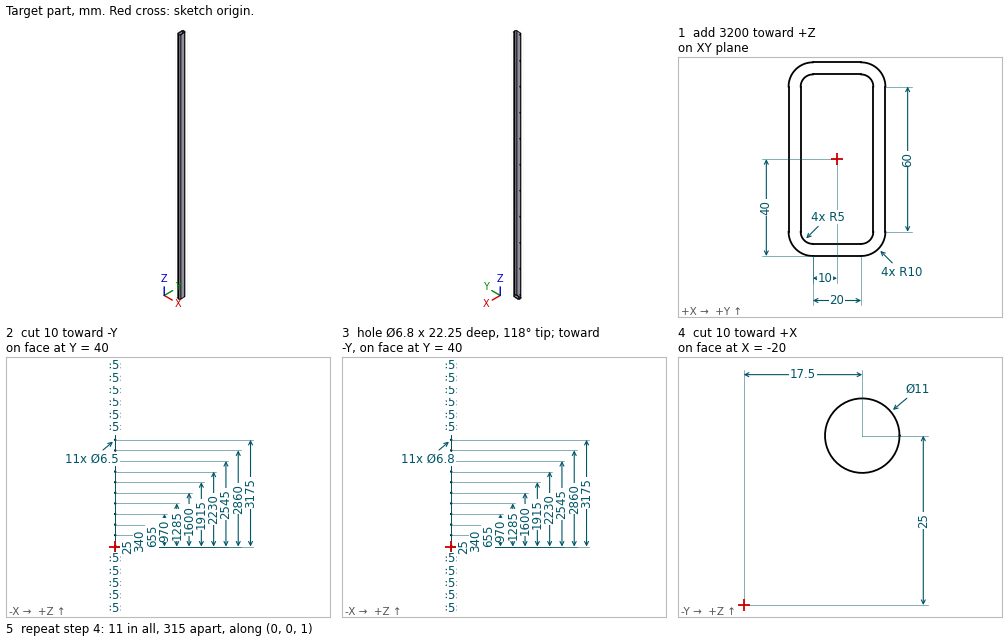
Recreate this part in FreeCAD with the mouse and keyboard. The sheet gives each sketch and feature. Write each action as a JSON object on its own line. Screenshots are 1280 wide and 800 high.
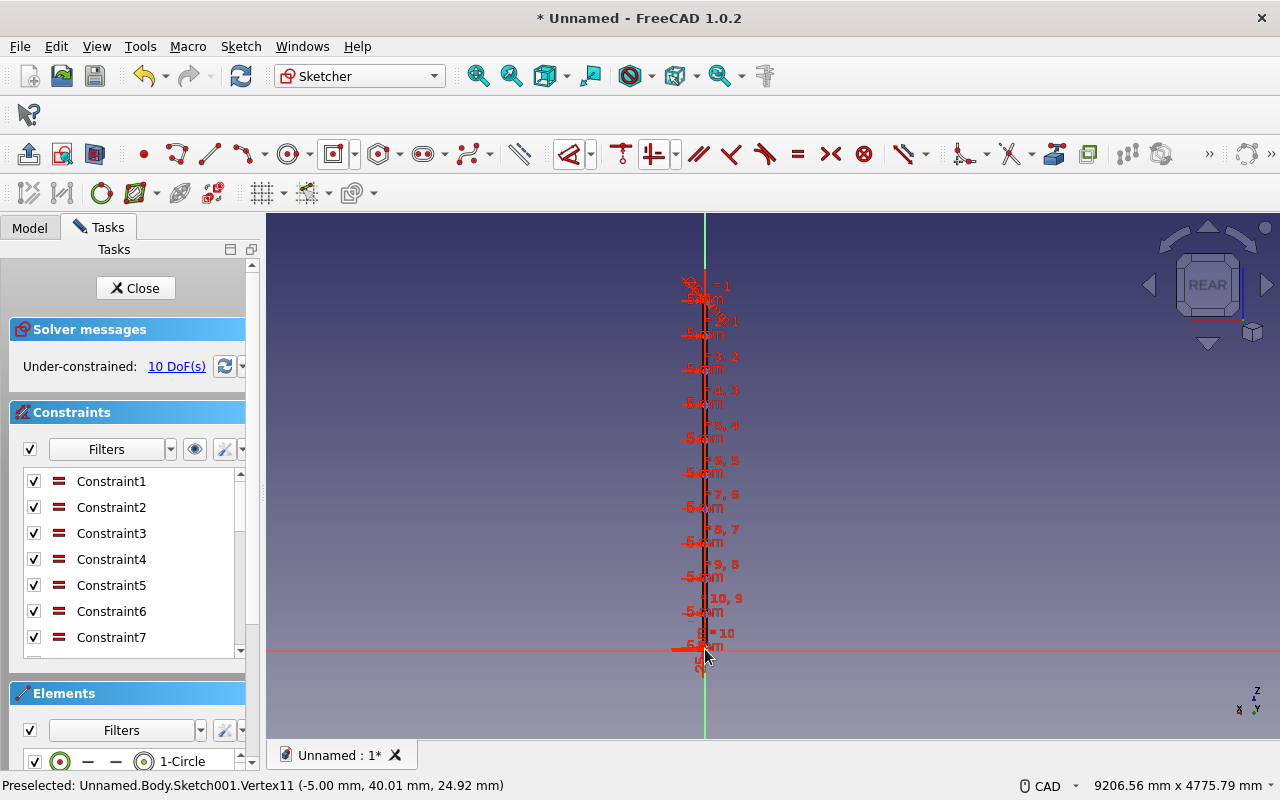
{"action": "left_click", "coordinate": [705, 545]}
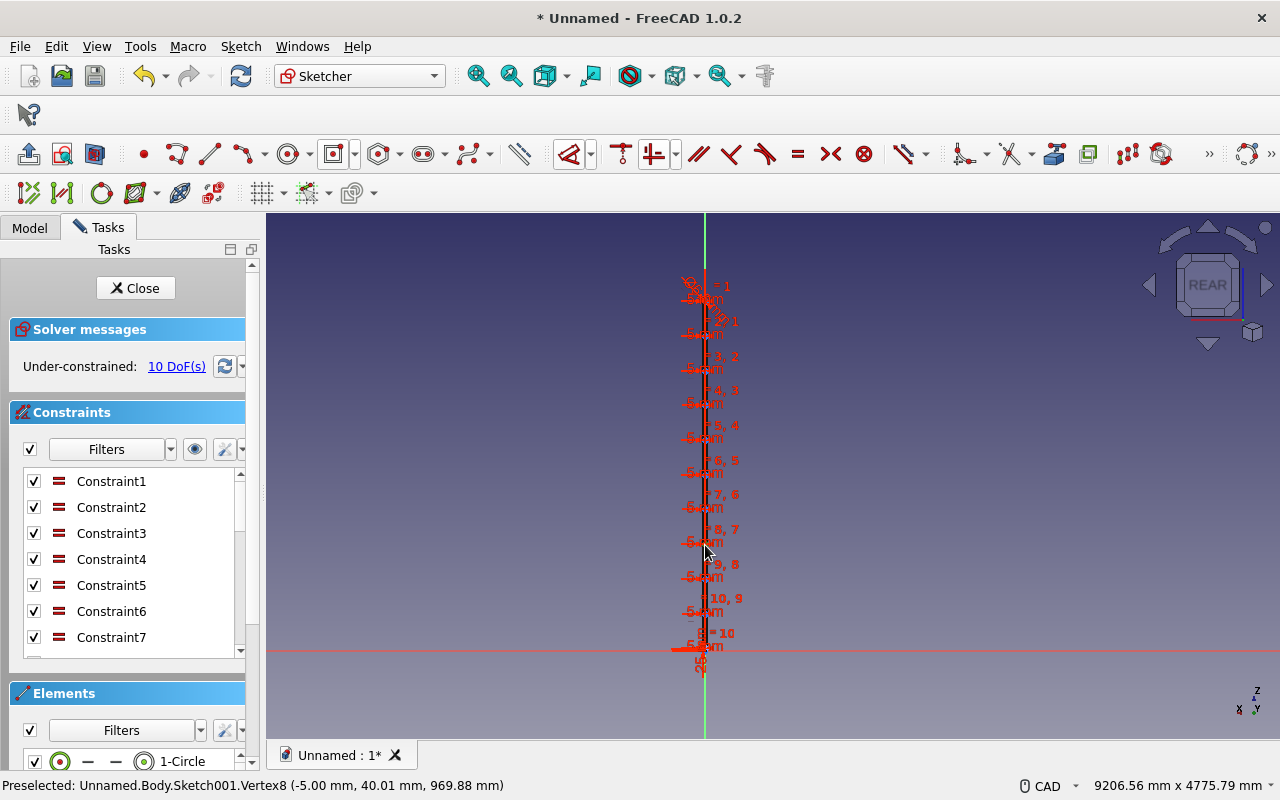
{"action": "left_click", "coordinate": [590, 154]}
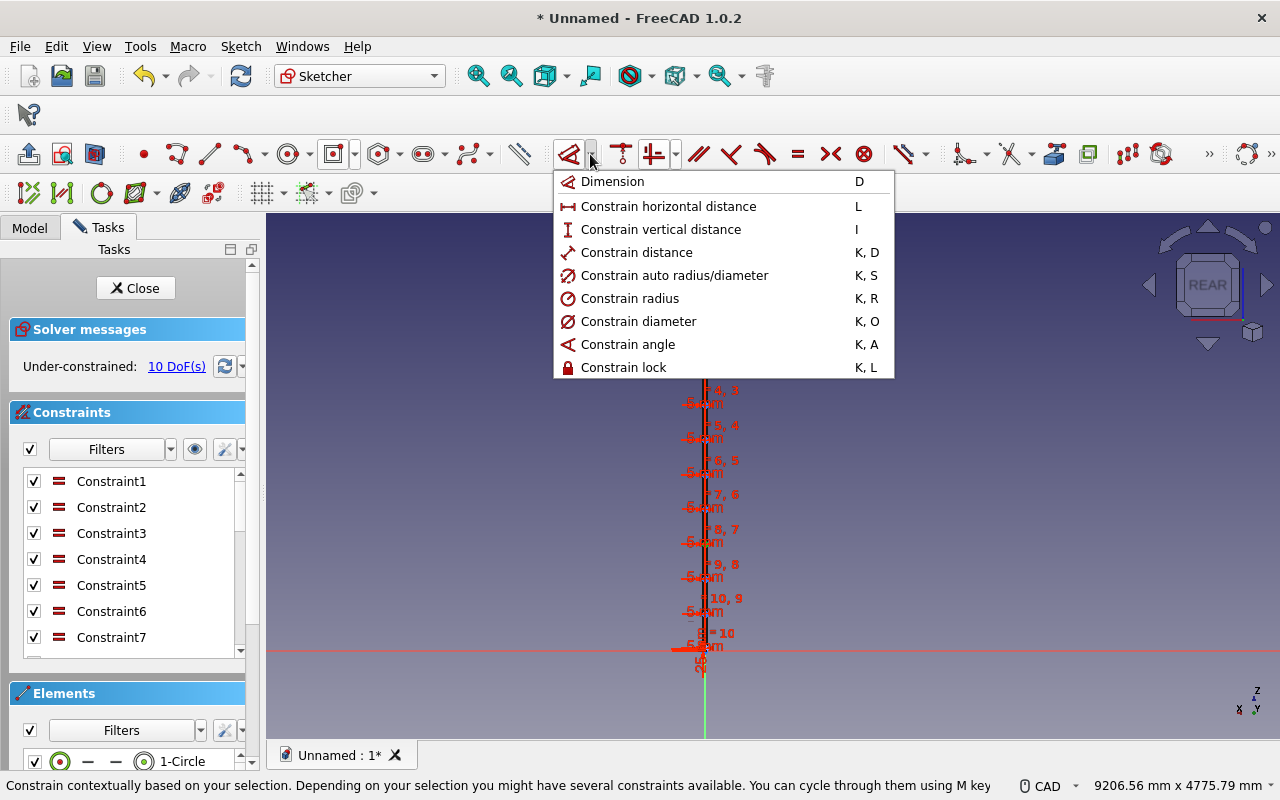
{"action": "left_click", "coordinate": [724, 230]}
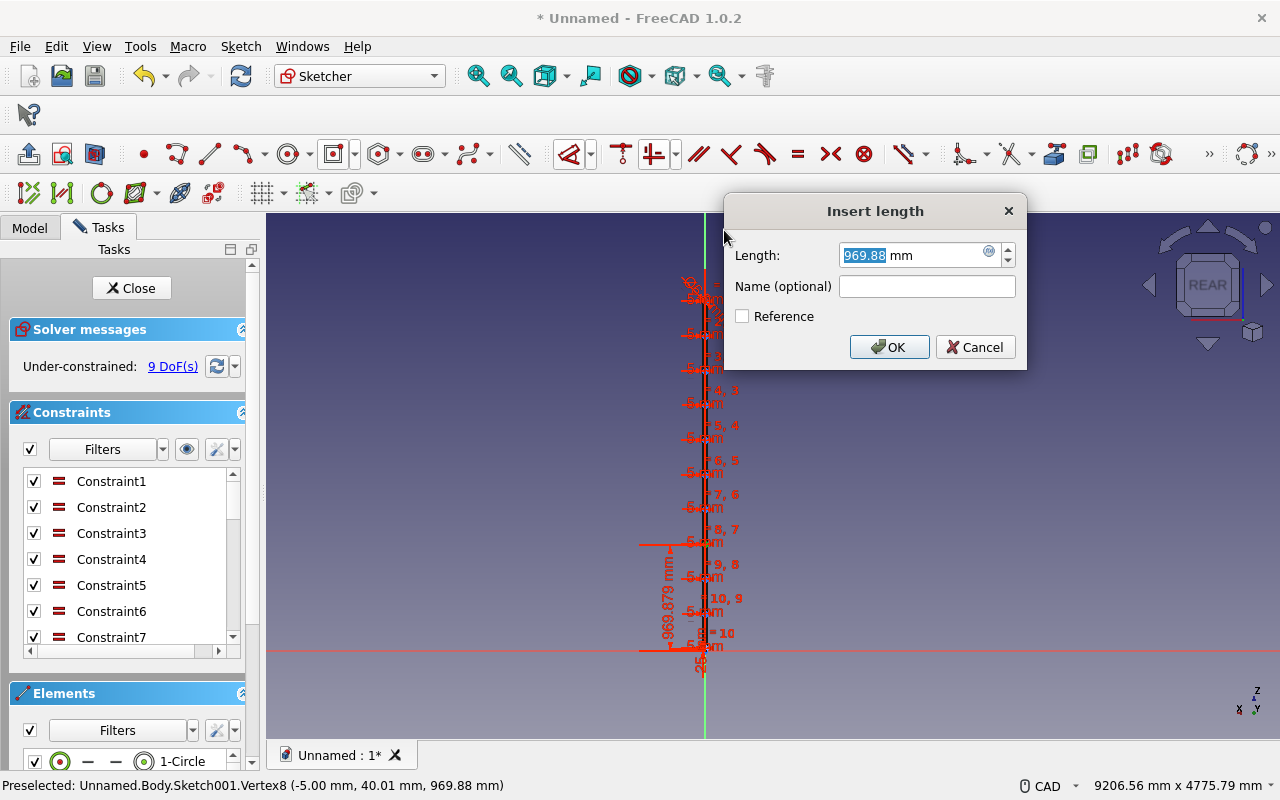
{"action": "type", "text": "970"}
{"action": "key", "text": "Return"}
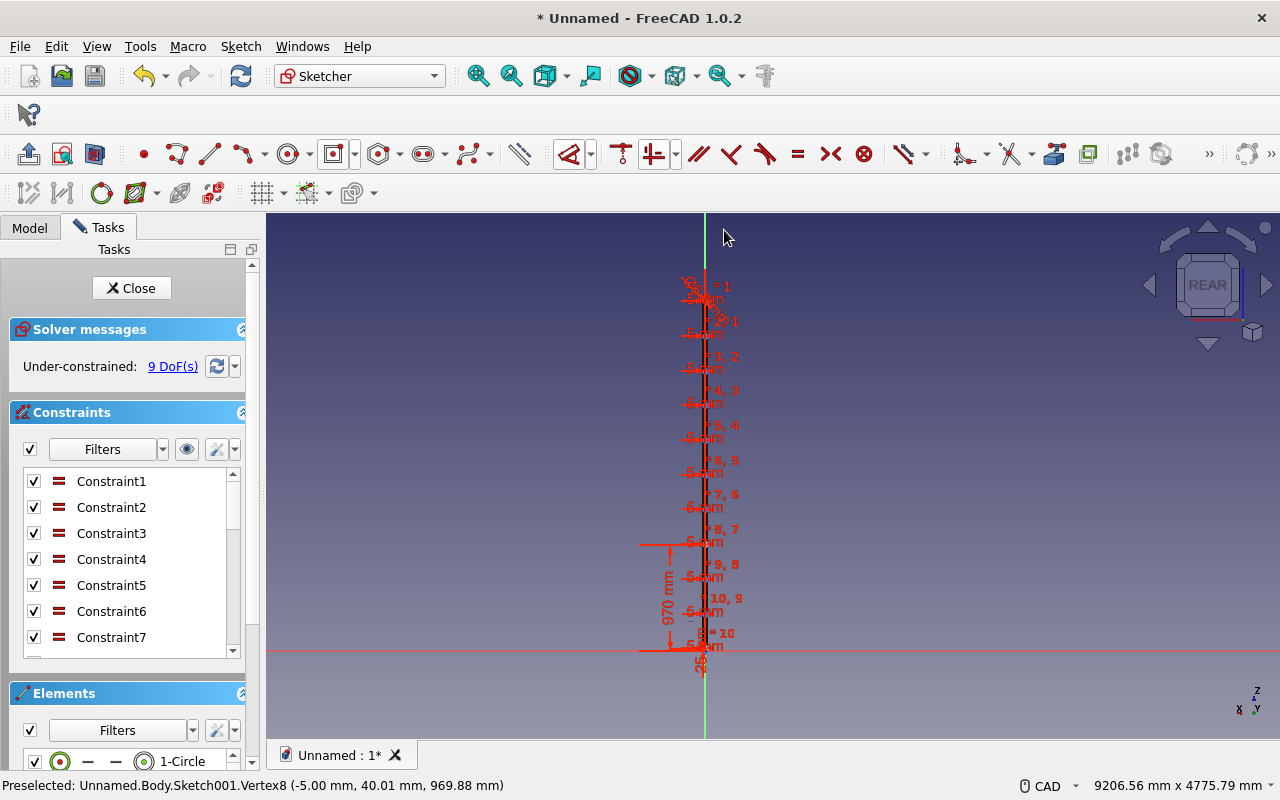
{"action": "left_click", "coordinate": [705, 579]}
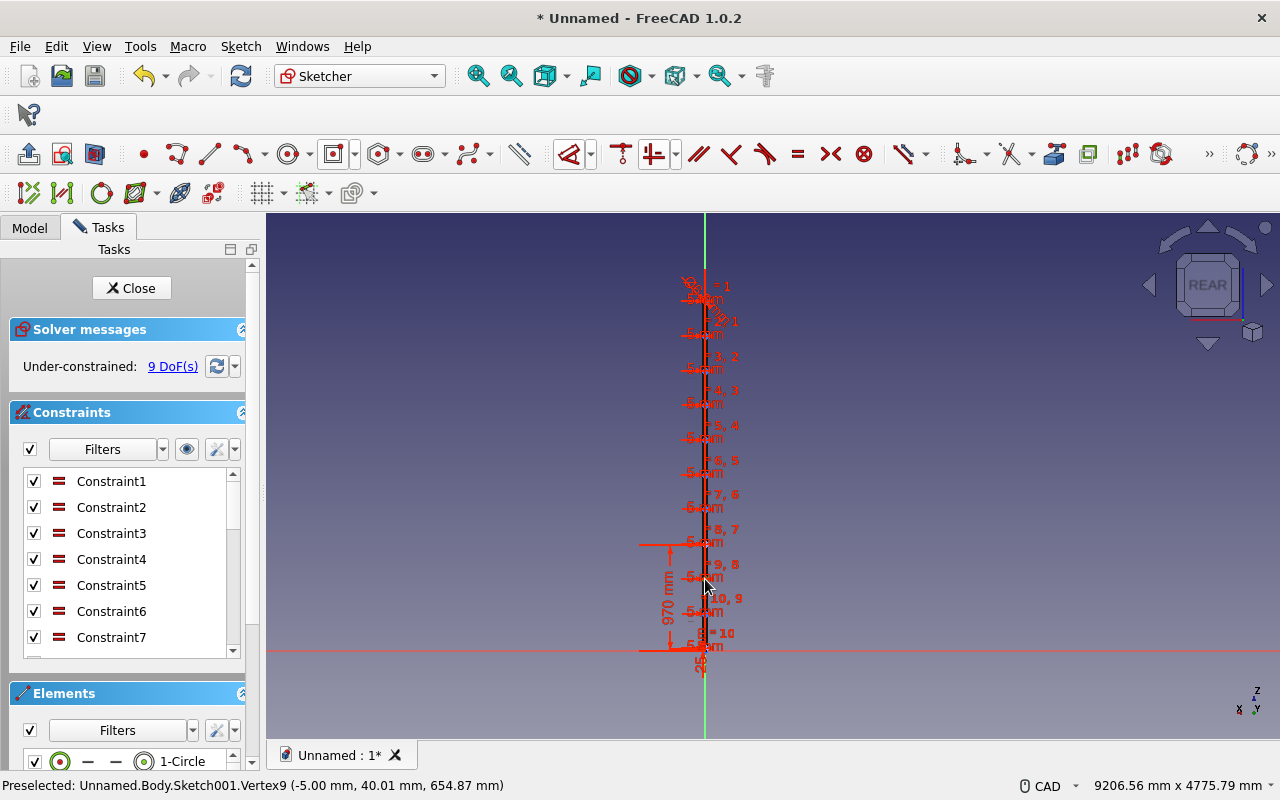
{"action": "left_click", "coordinate": [590, 154]}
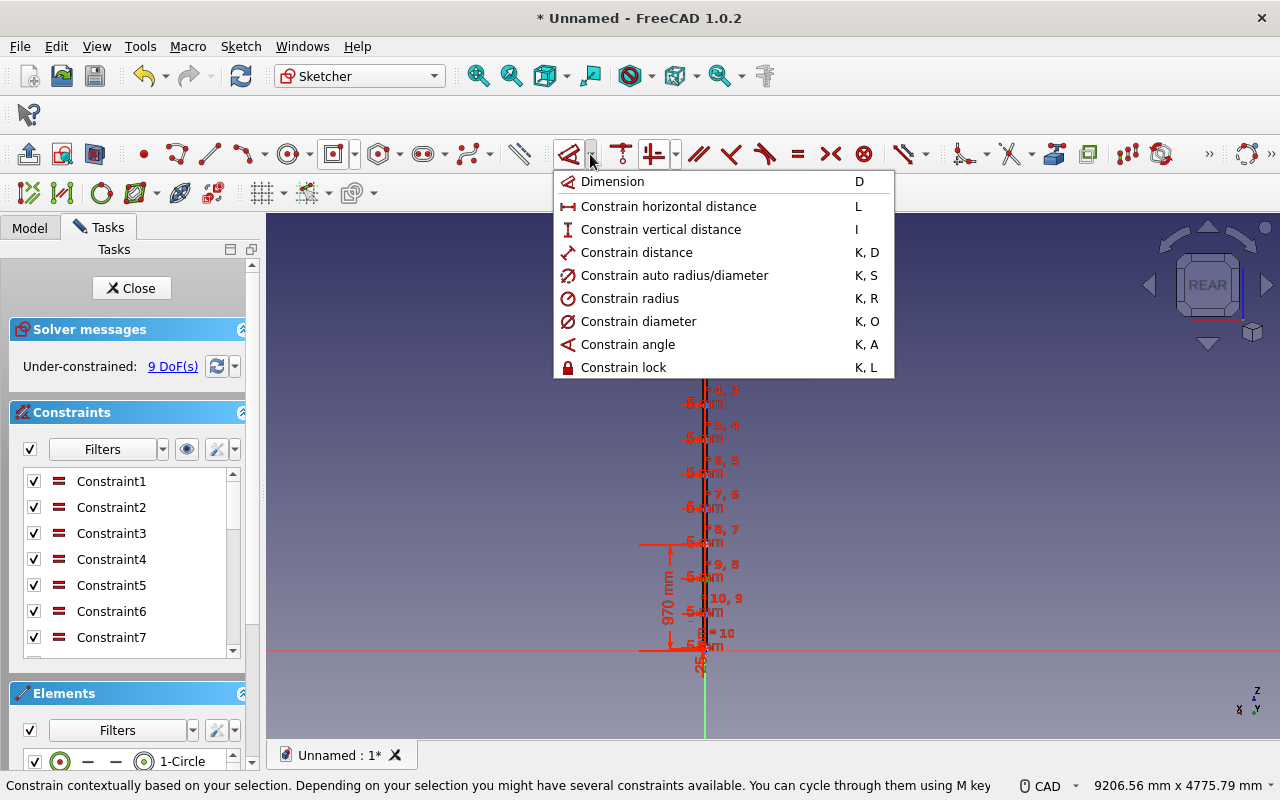
{"action": "left_click", "coordinate": [724, 230]}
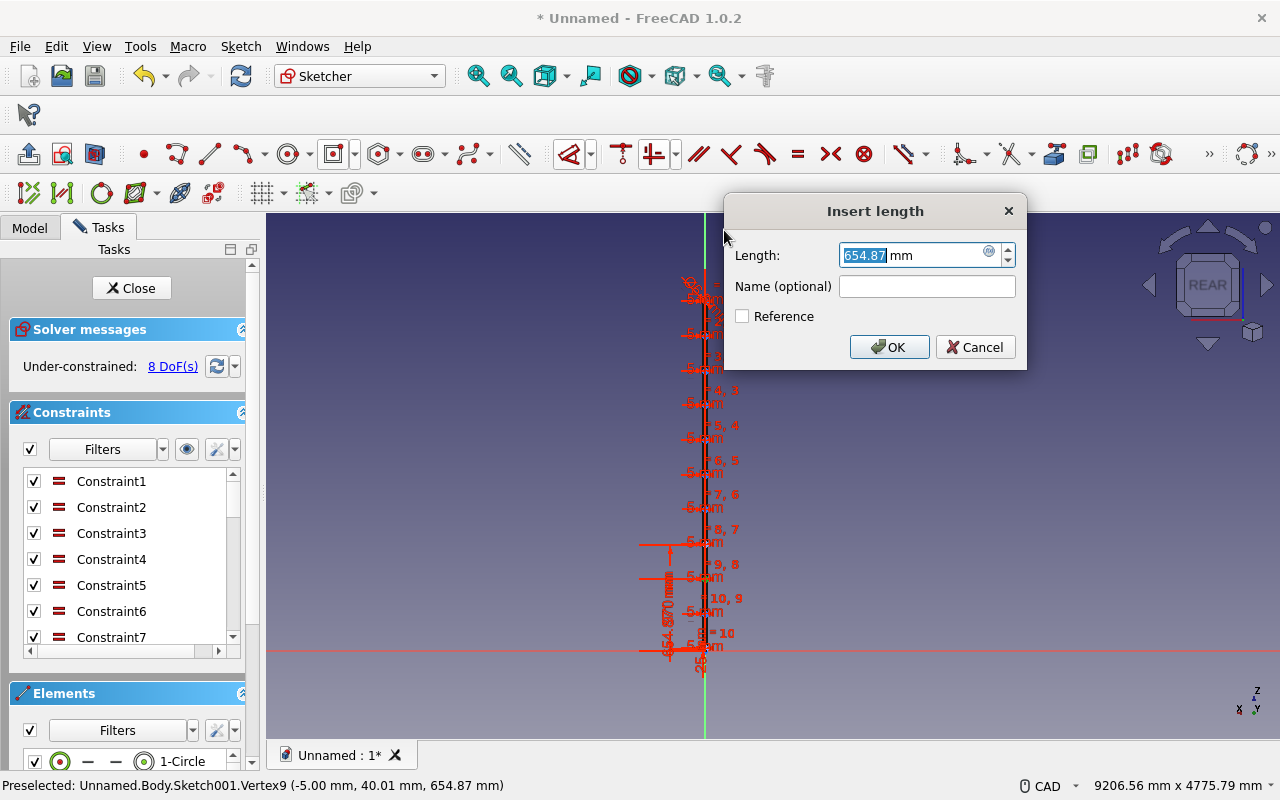
{"action": "type", "text": "655"}
{"action": "key", "text": "Return"}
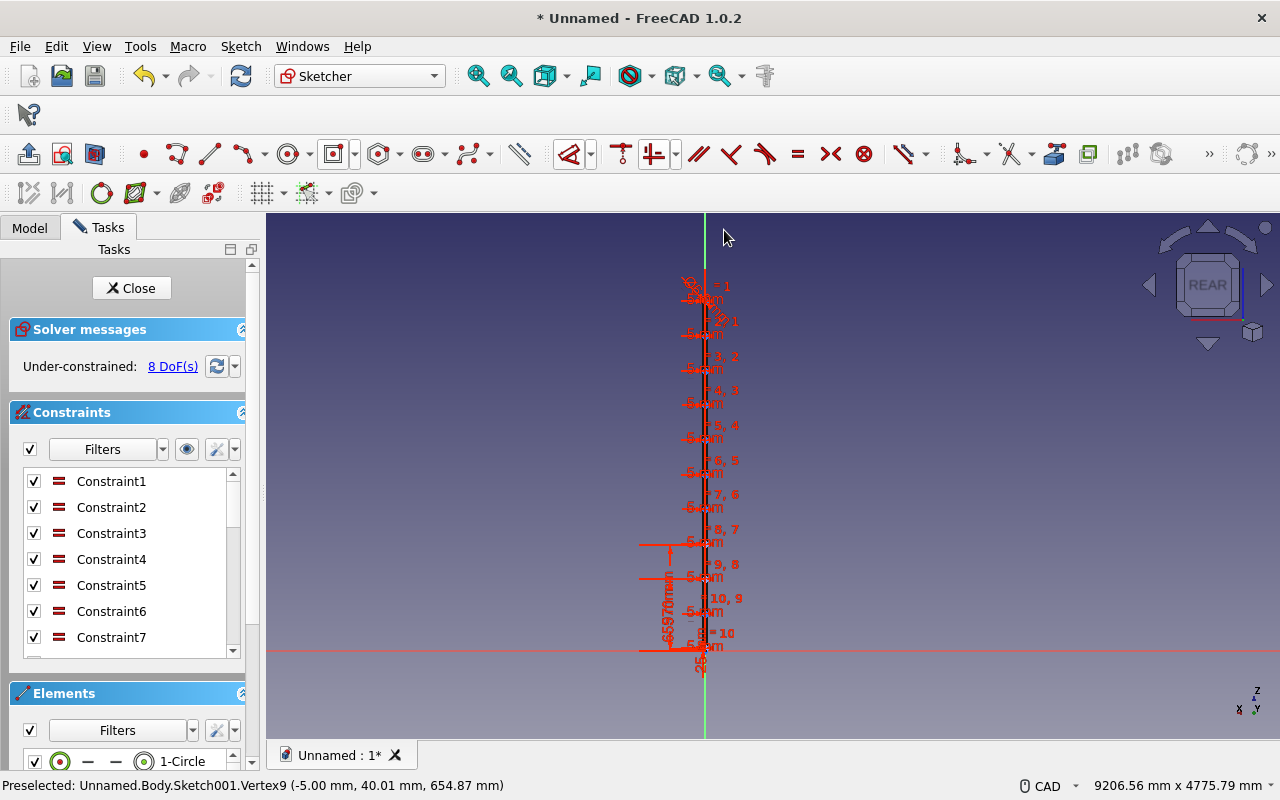
{"action": "left_click", "coordinate": [705, 614]}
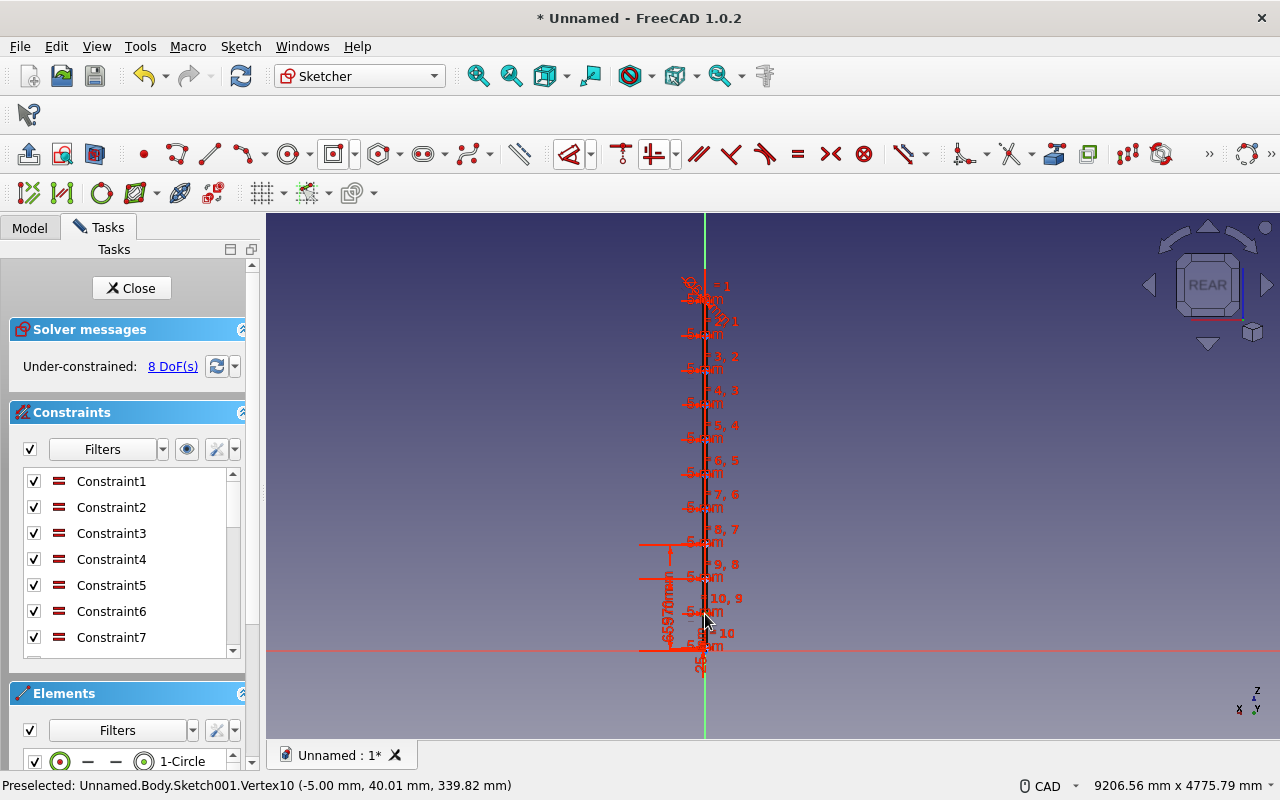
{"action": "key", "text": "i"}